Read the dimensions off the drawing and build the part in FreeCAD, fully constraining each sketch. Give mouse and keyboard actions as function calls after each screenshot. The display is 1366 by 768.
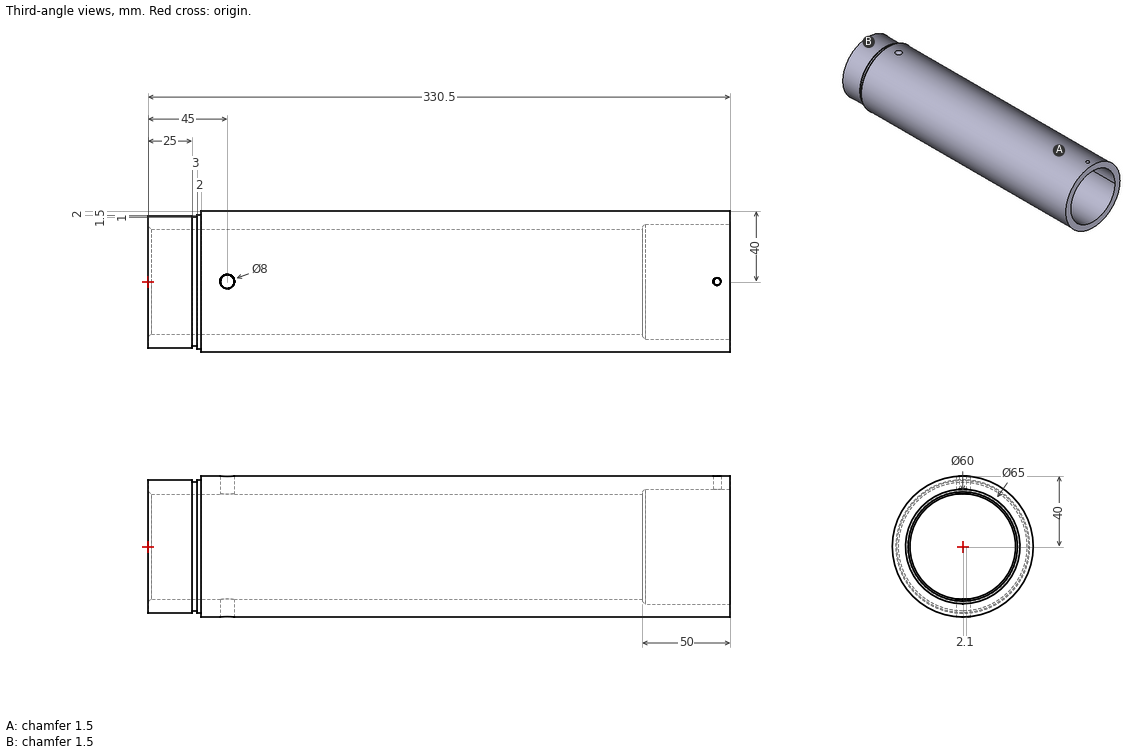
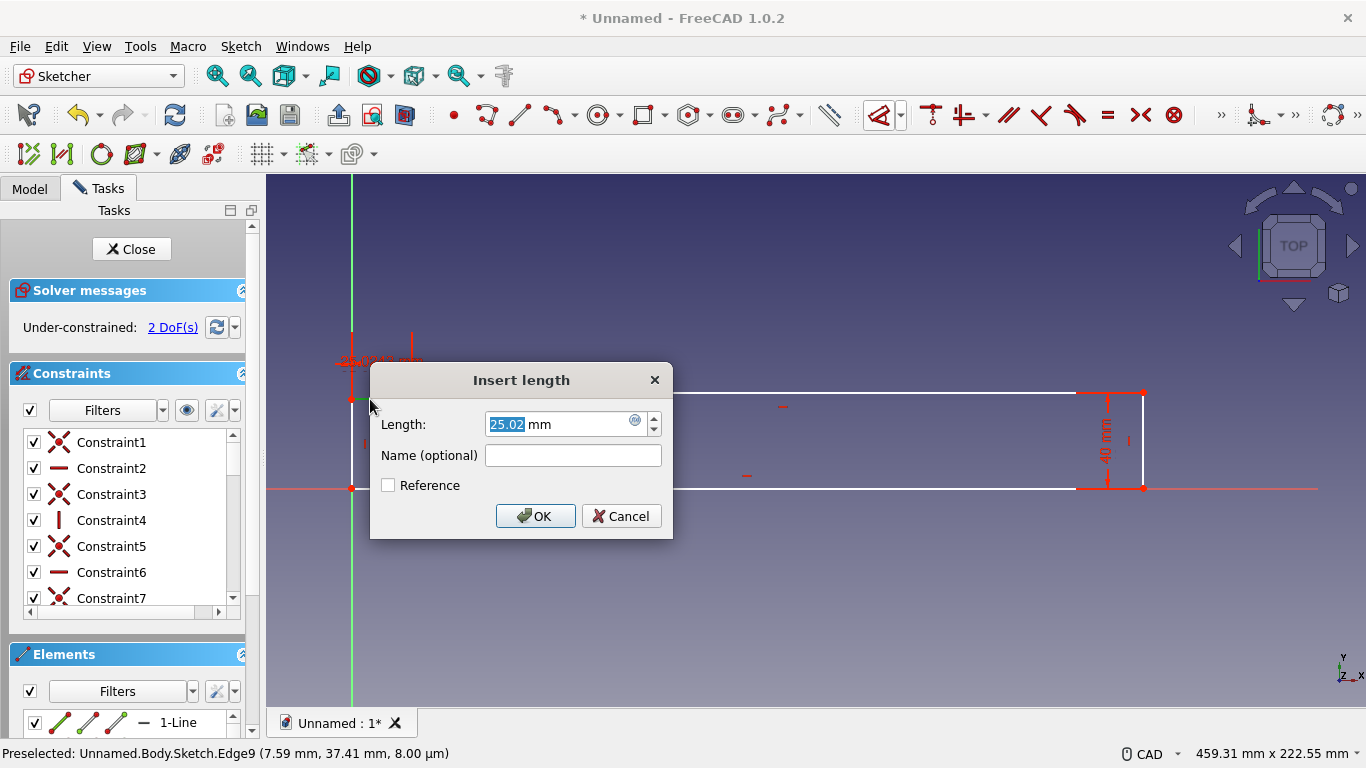
text(25)
key(Return)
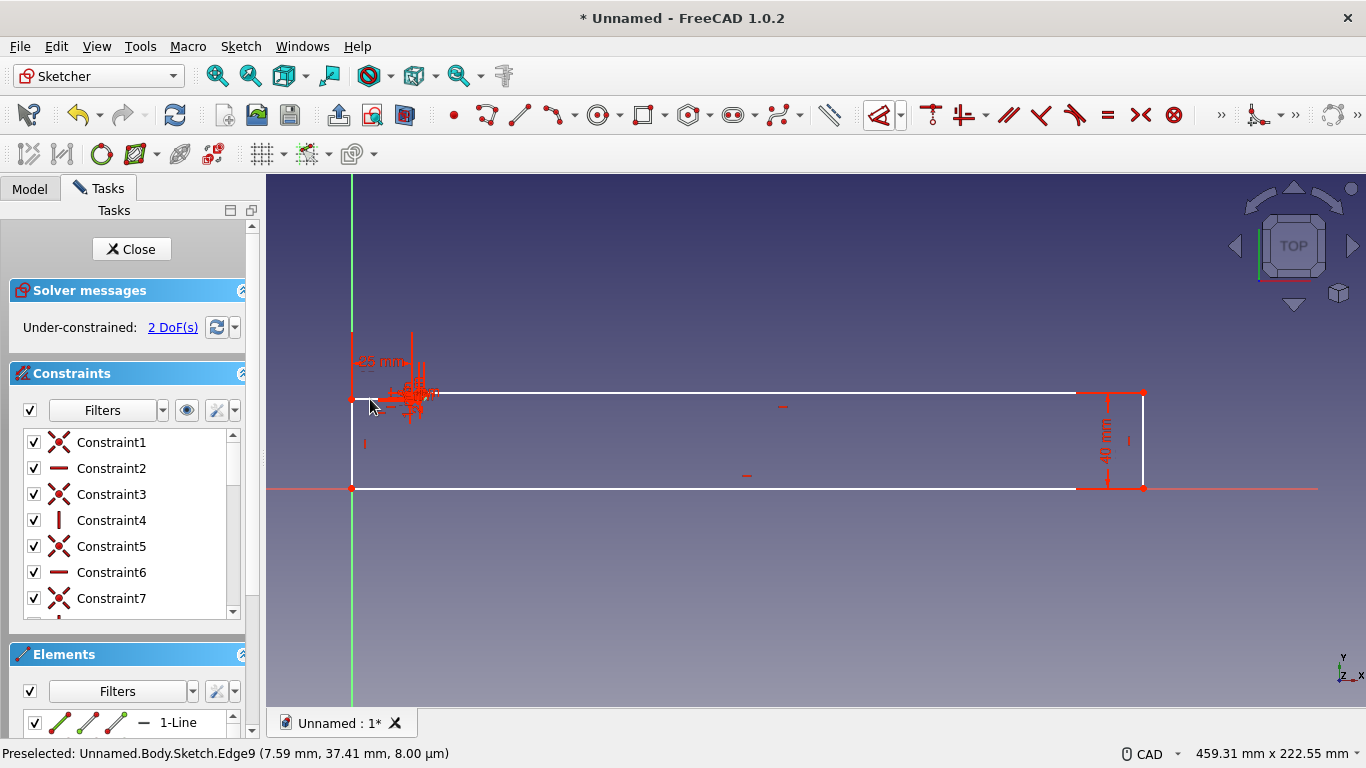
scroll(419, 400, up, 13)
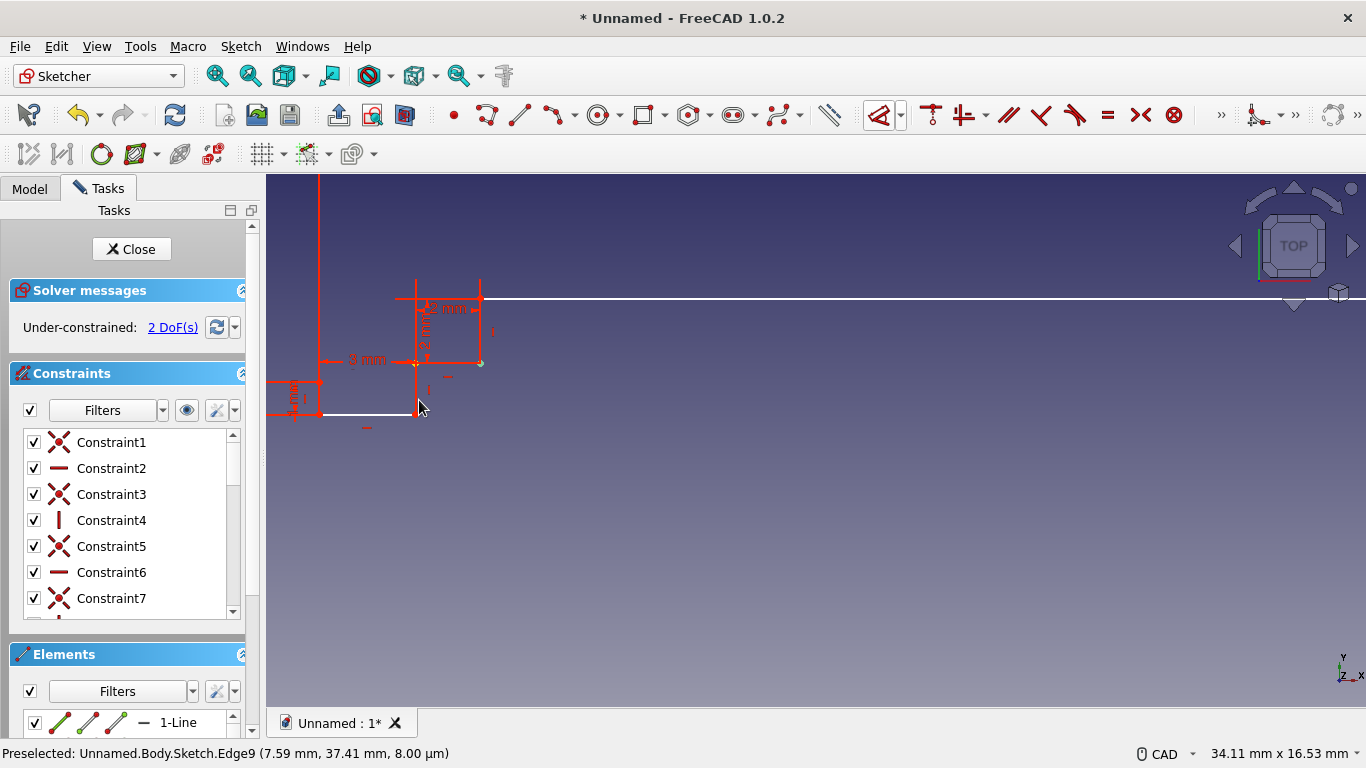
click(416, 389)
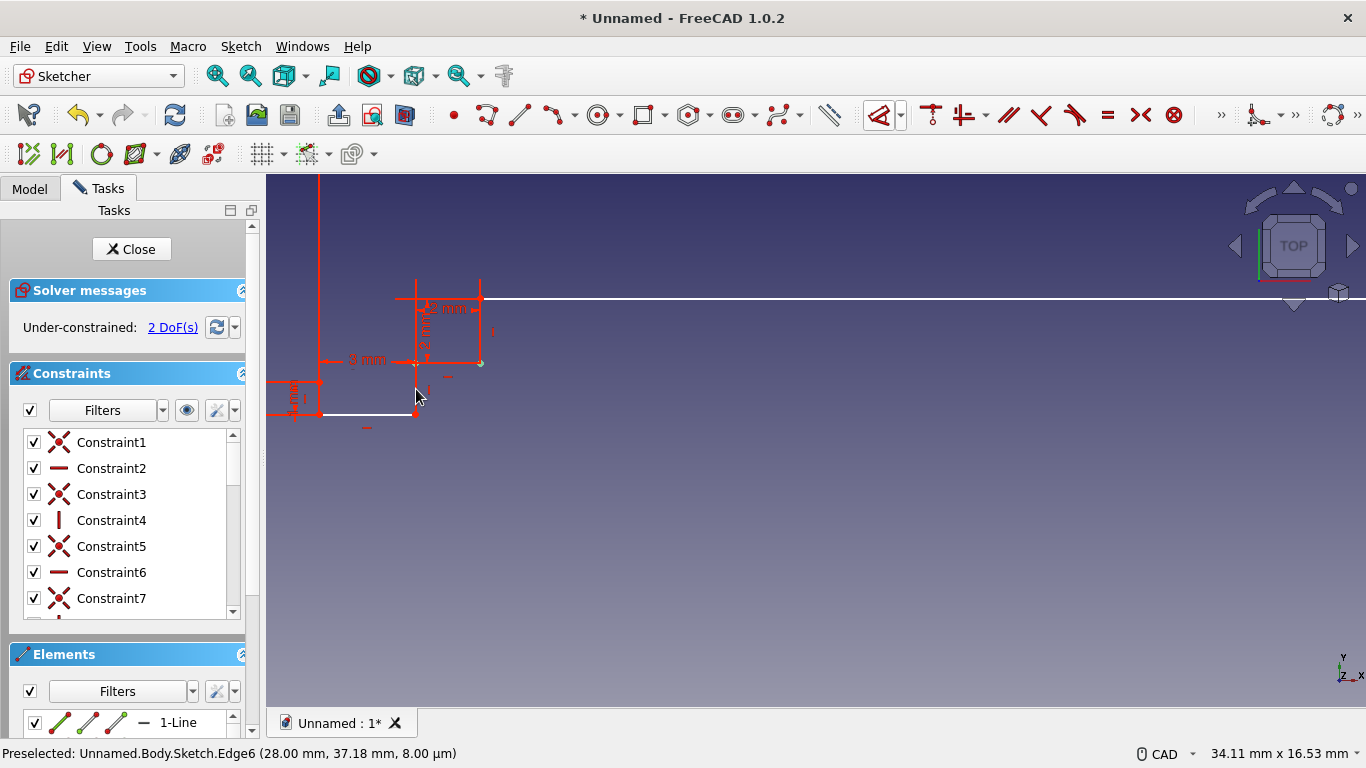
click(900, 116)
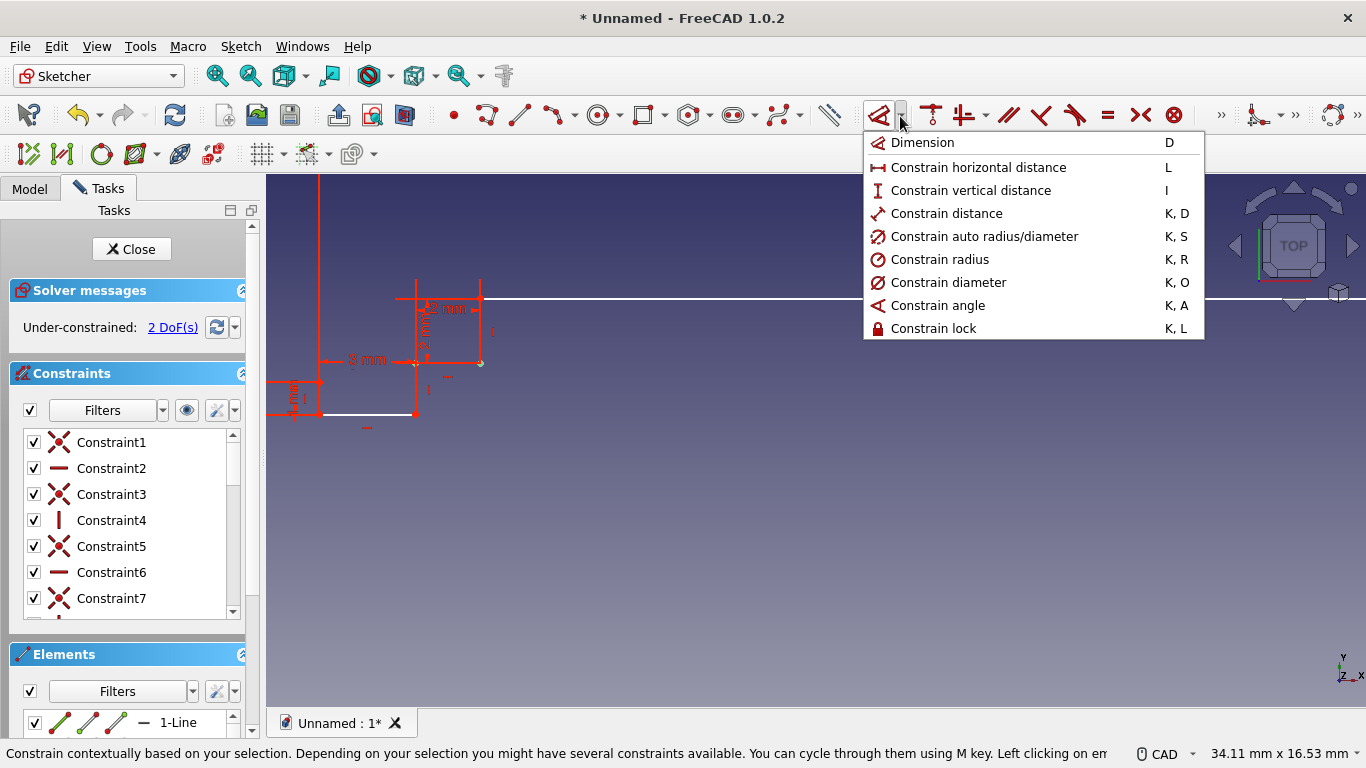
click(1034, 190)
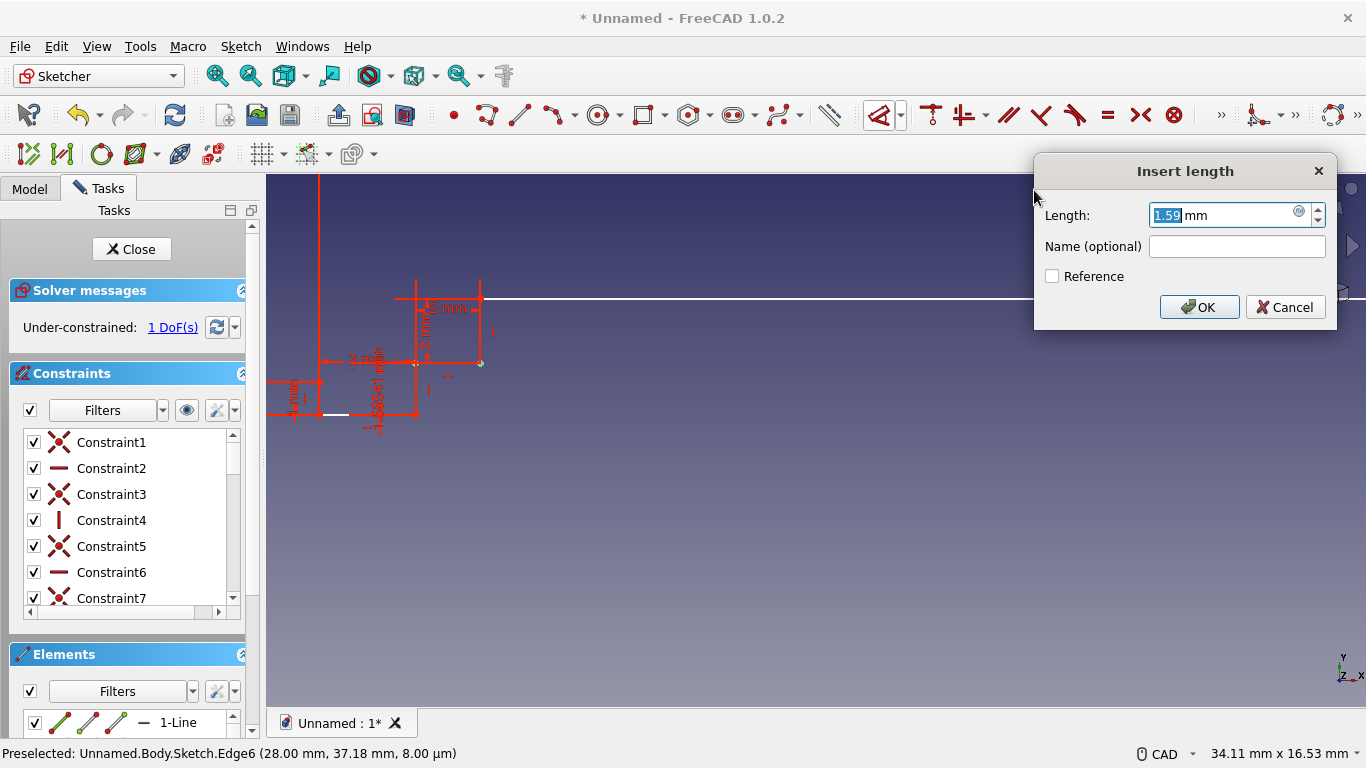
text(1.5)
key(Return)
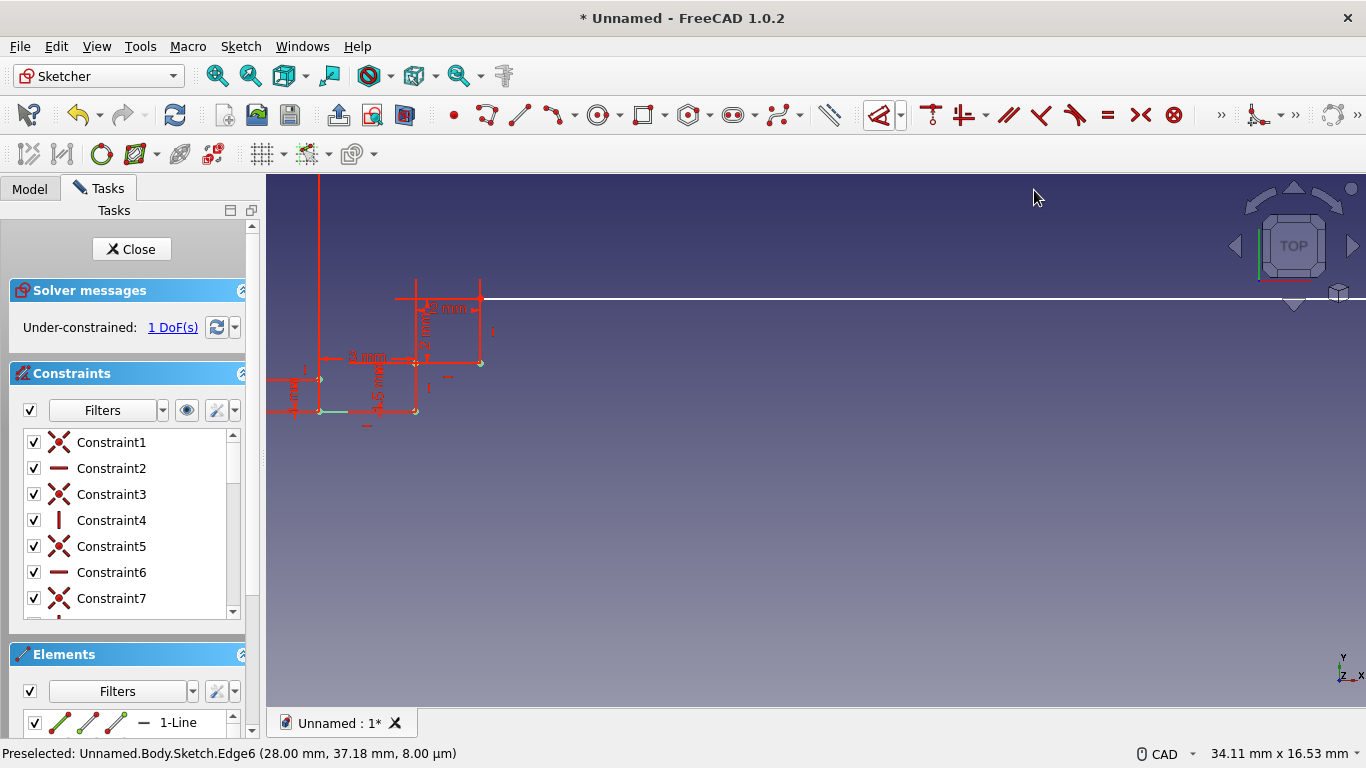
scroll(482, 408, down, 14)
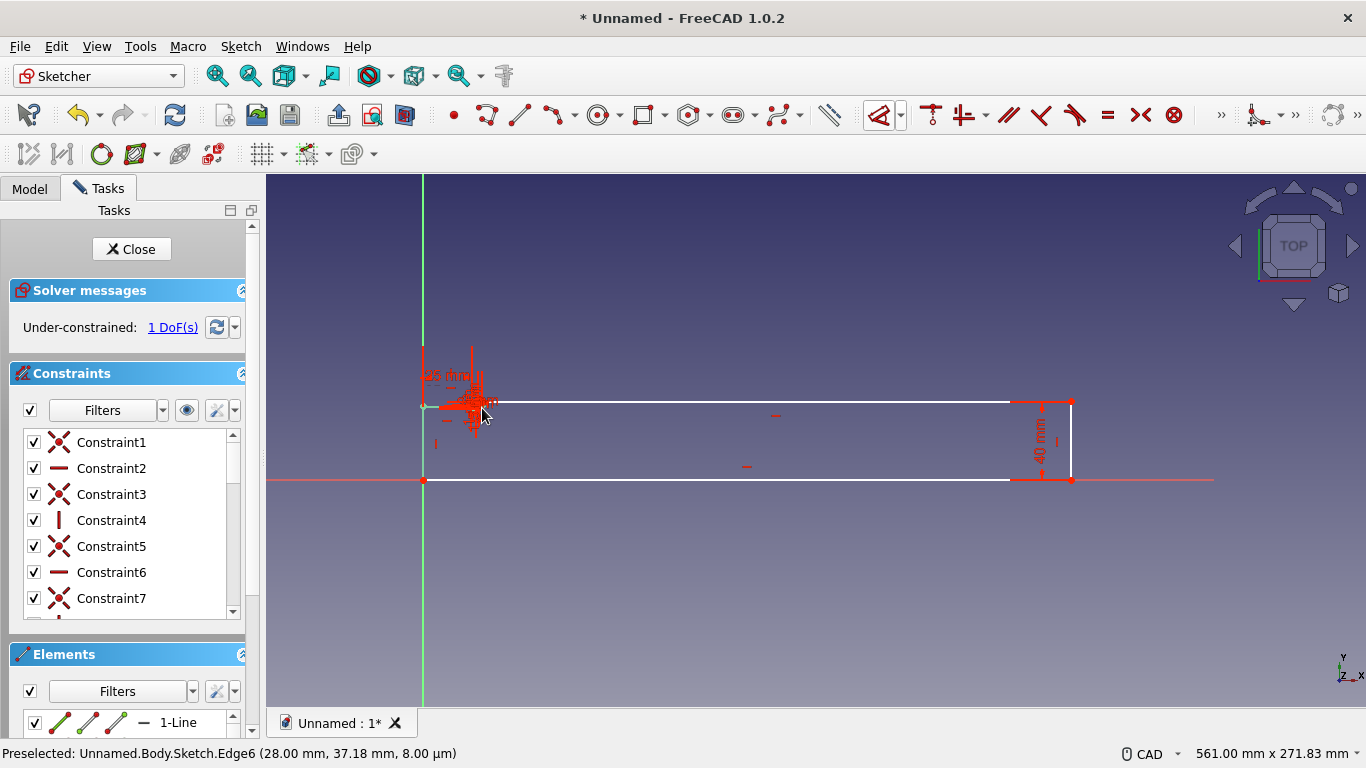
click(618, 480)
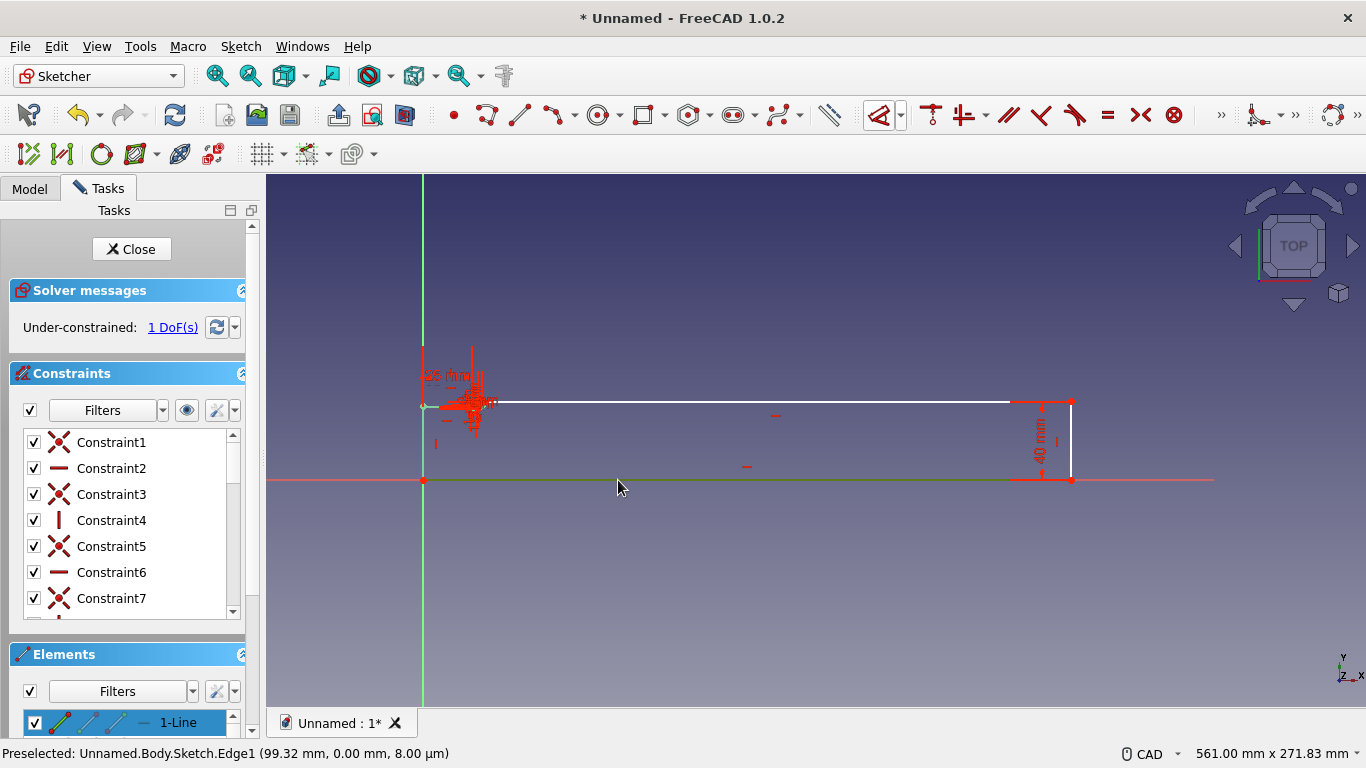
key(l)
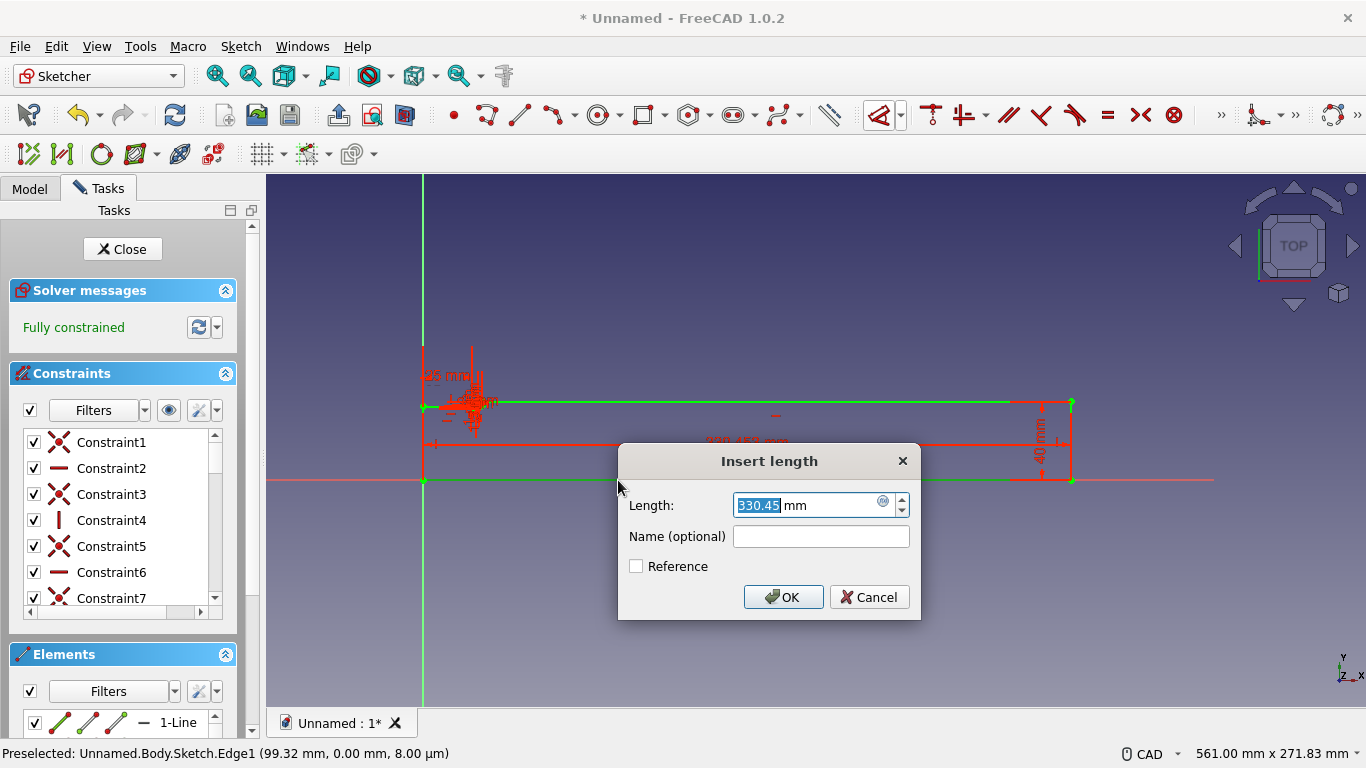
text(330.5)
key(Return)